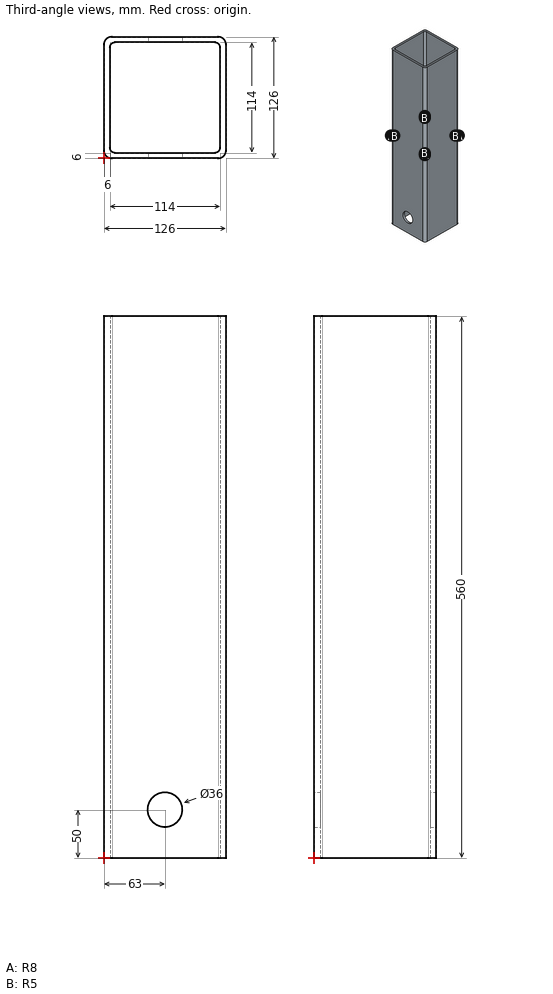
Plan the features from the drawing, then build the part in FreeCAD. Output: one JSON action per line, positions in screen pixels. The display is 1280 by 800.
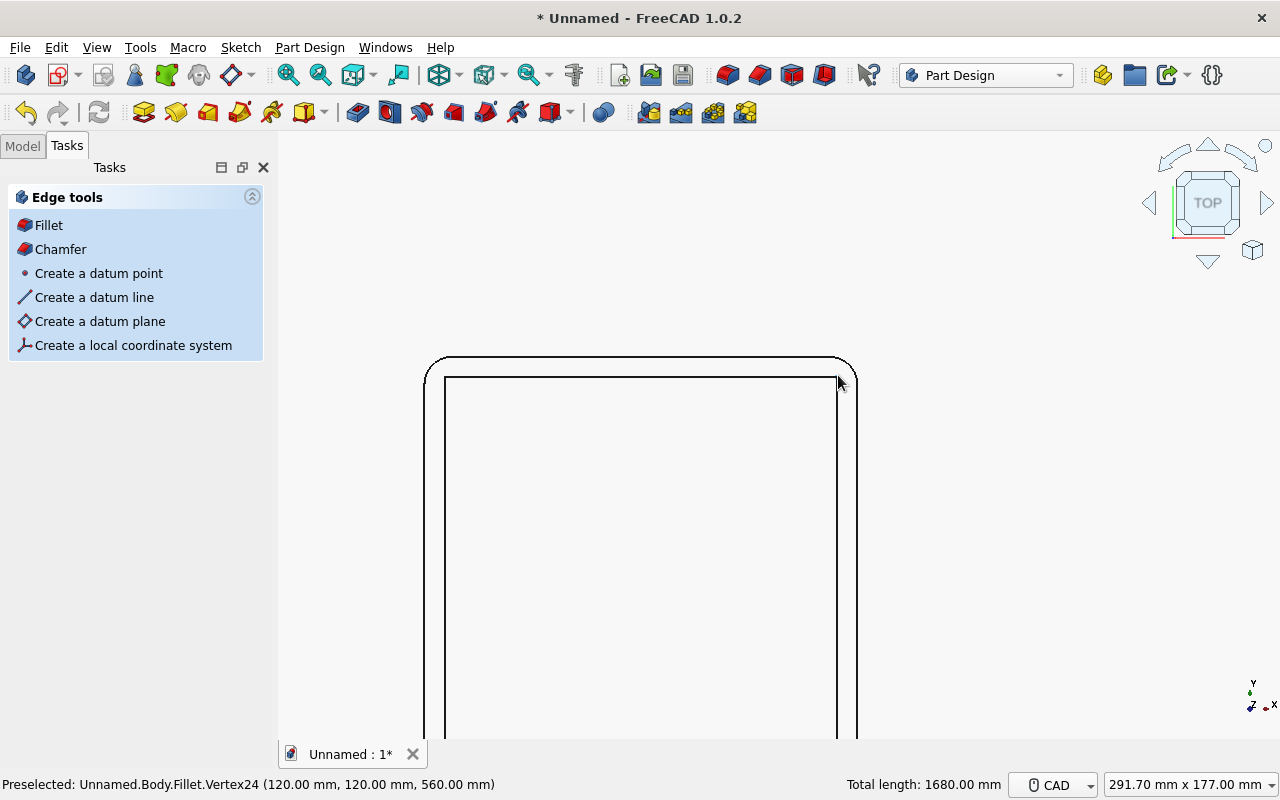
{"action": "left_click", "coordinate": [290, 76]}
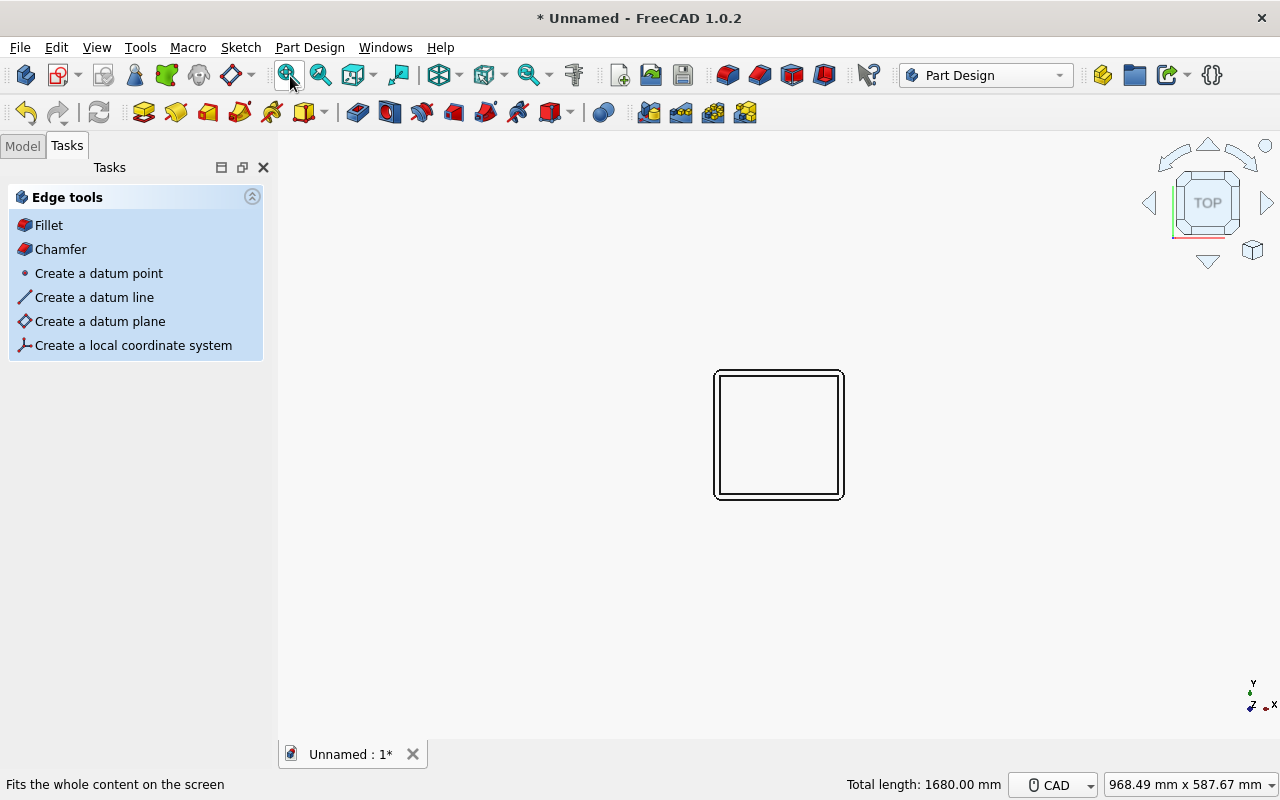
{"action": "key", "text": "1"}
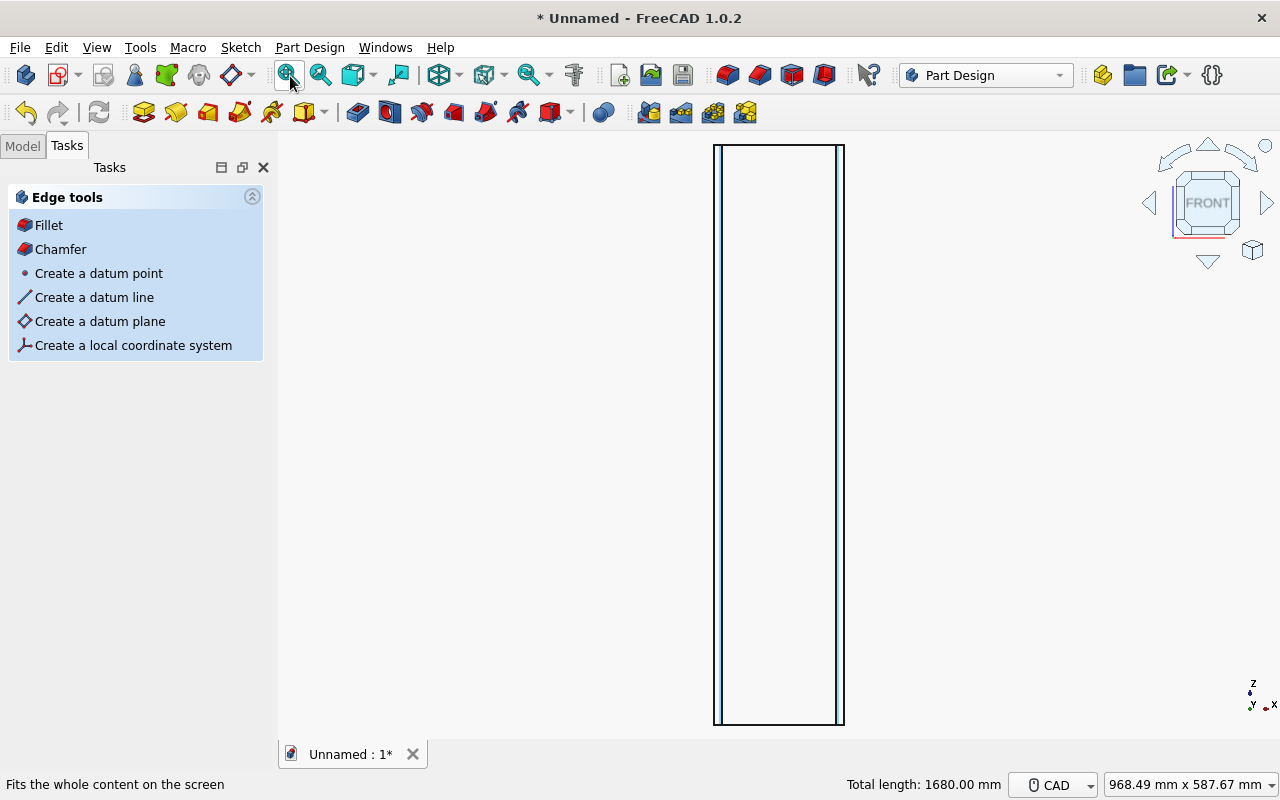
{"action": "scroll", "coordinate": [838, 434], "scroll_direction": "up", "scroll_amount": 6}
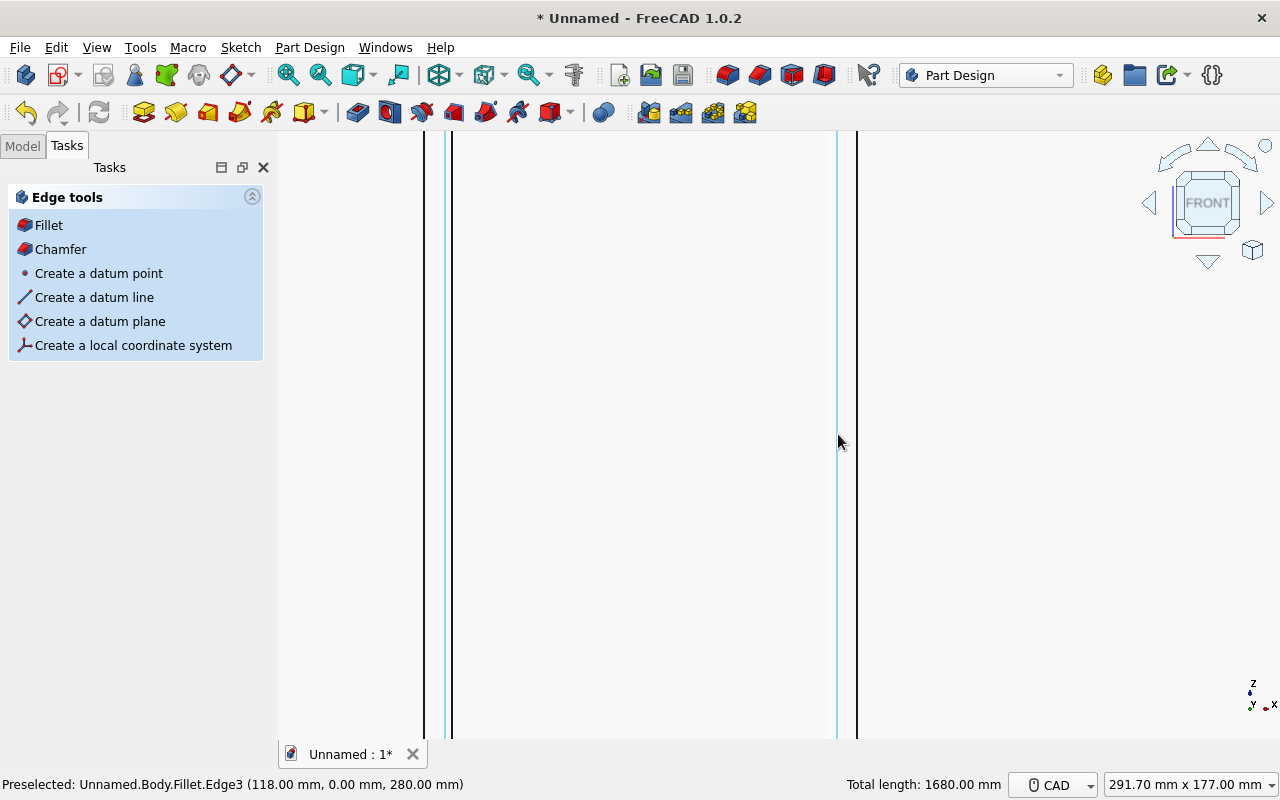
{"action": "left_click", "coordinate": [290, 76]}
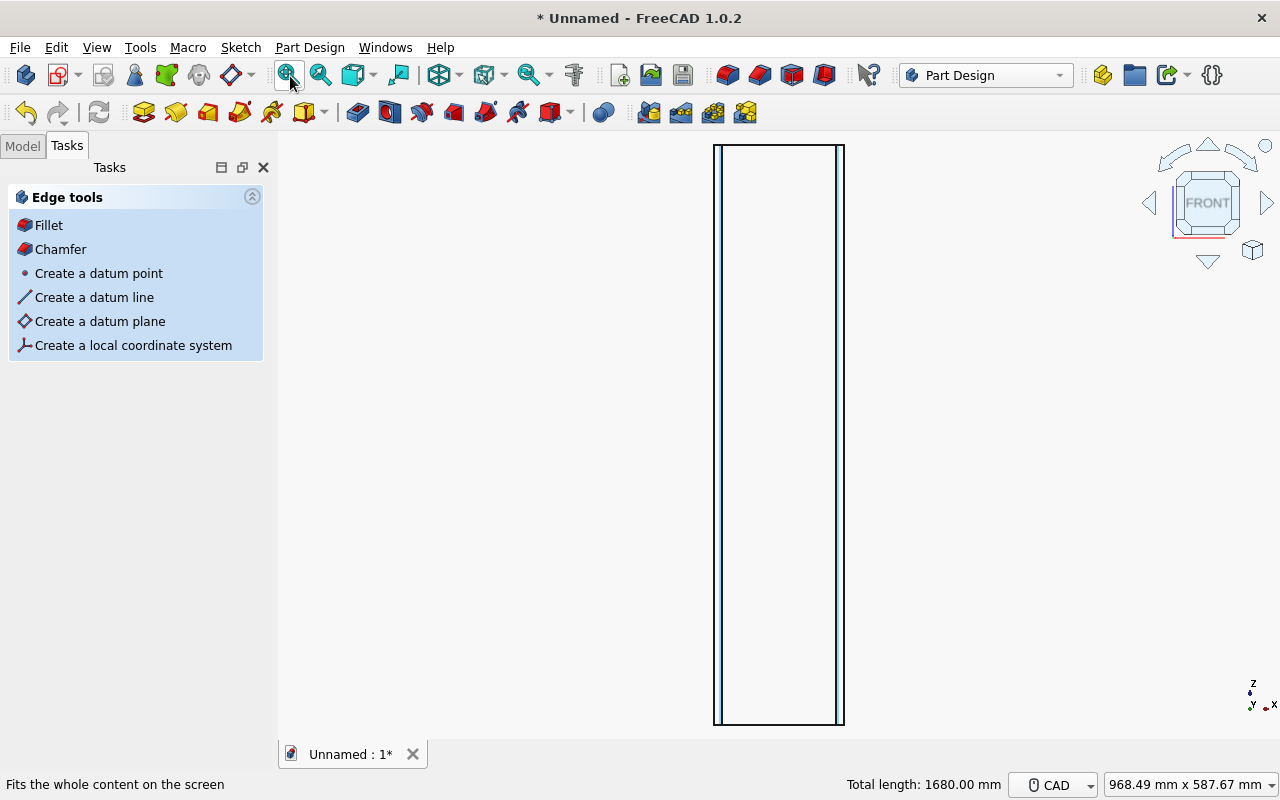
{"action": "key", "text": "3"}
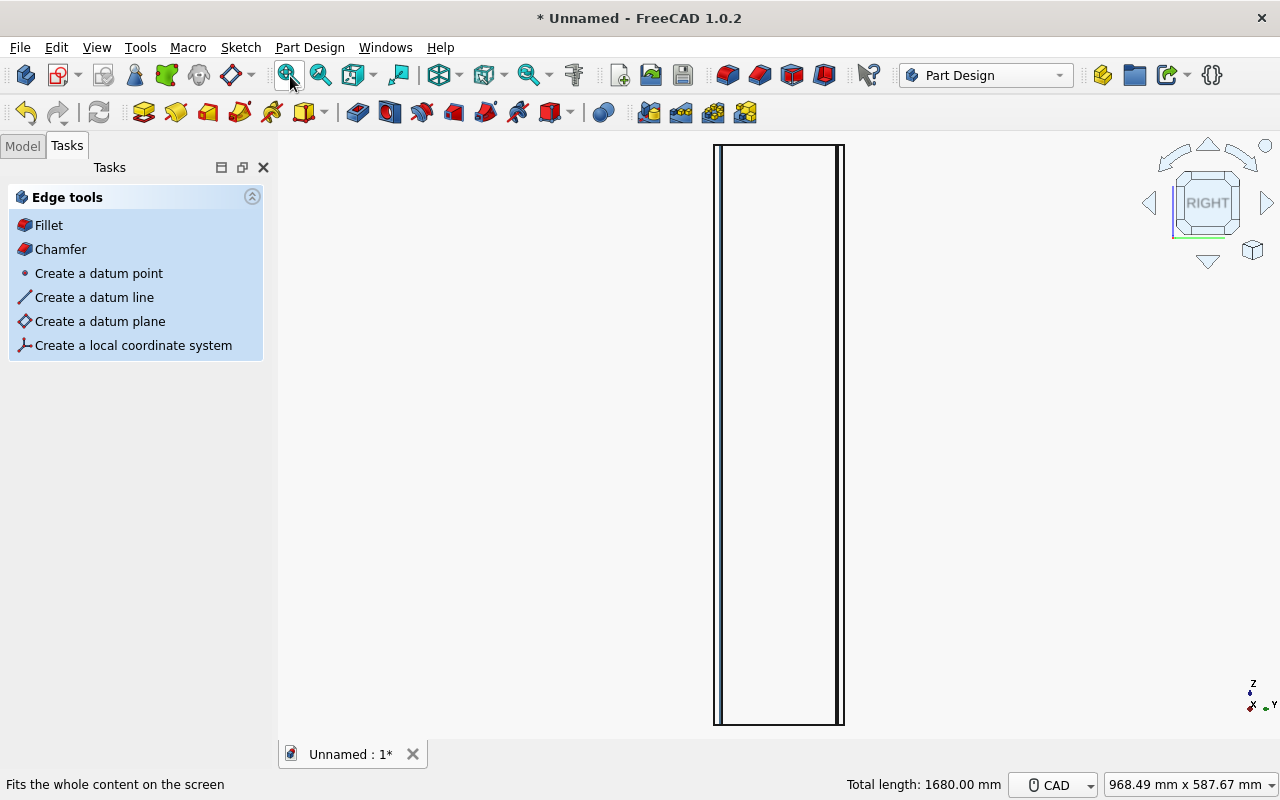
{"action": "scroll", "coordinate": [838, 434], "scroll_direction": "up", "scroll_amount": 6}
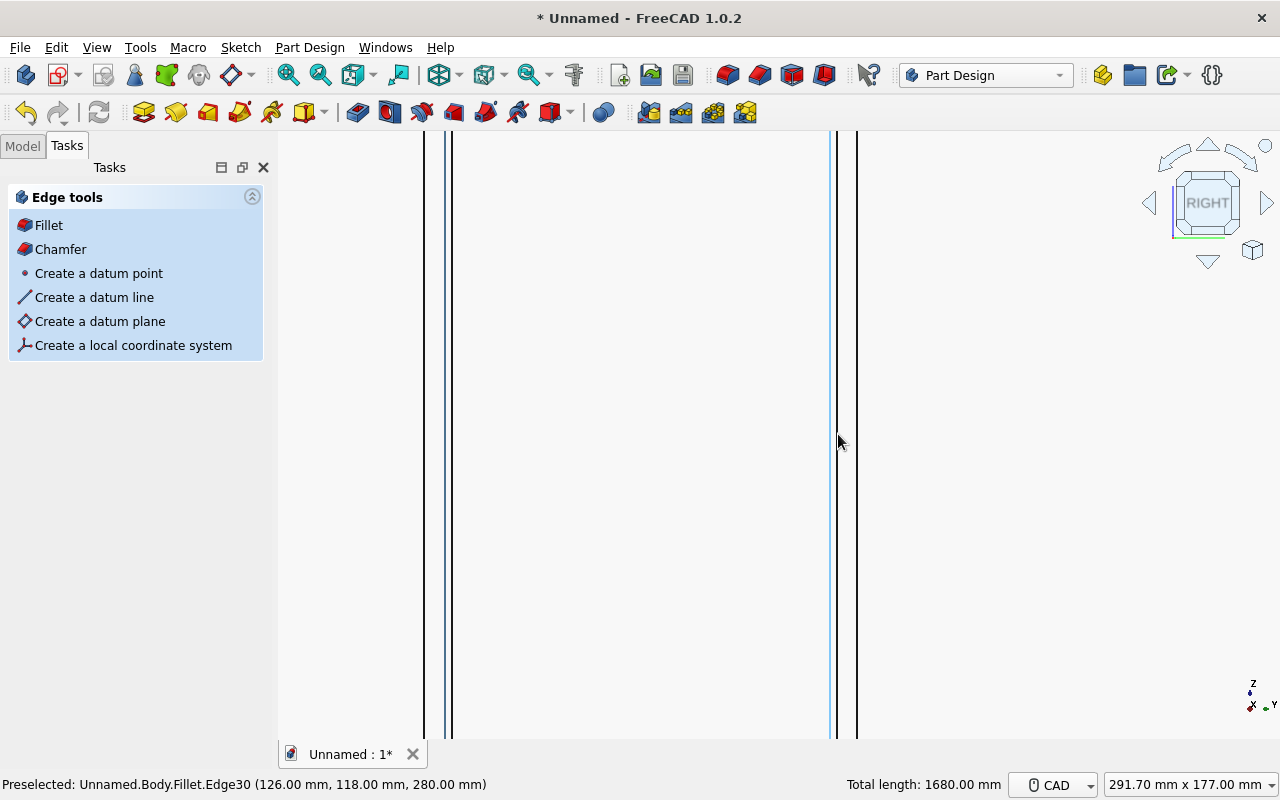
{"action": "left_click", "coordinate": [837, 435], "text": "ctrl"}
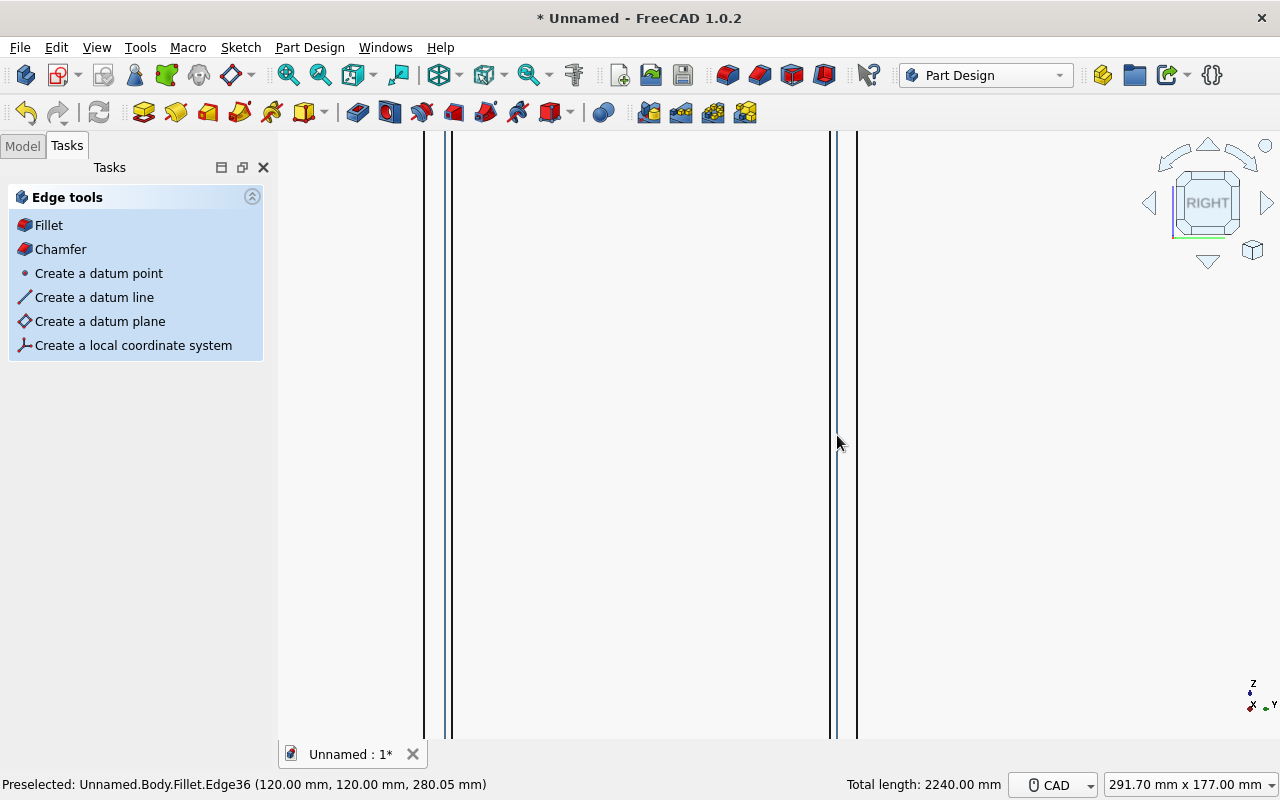
{"action": "key", "text": "v 1"}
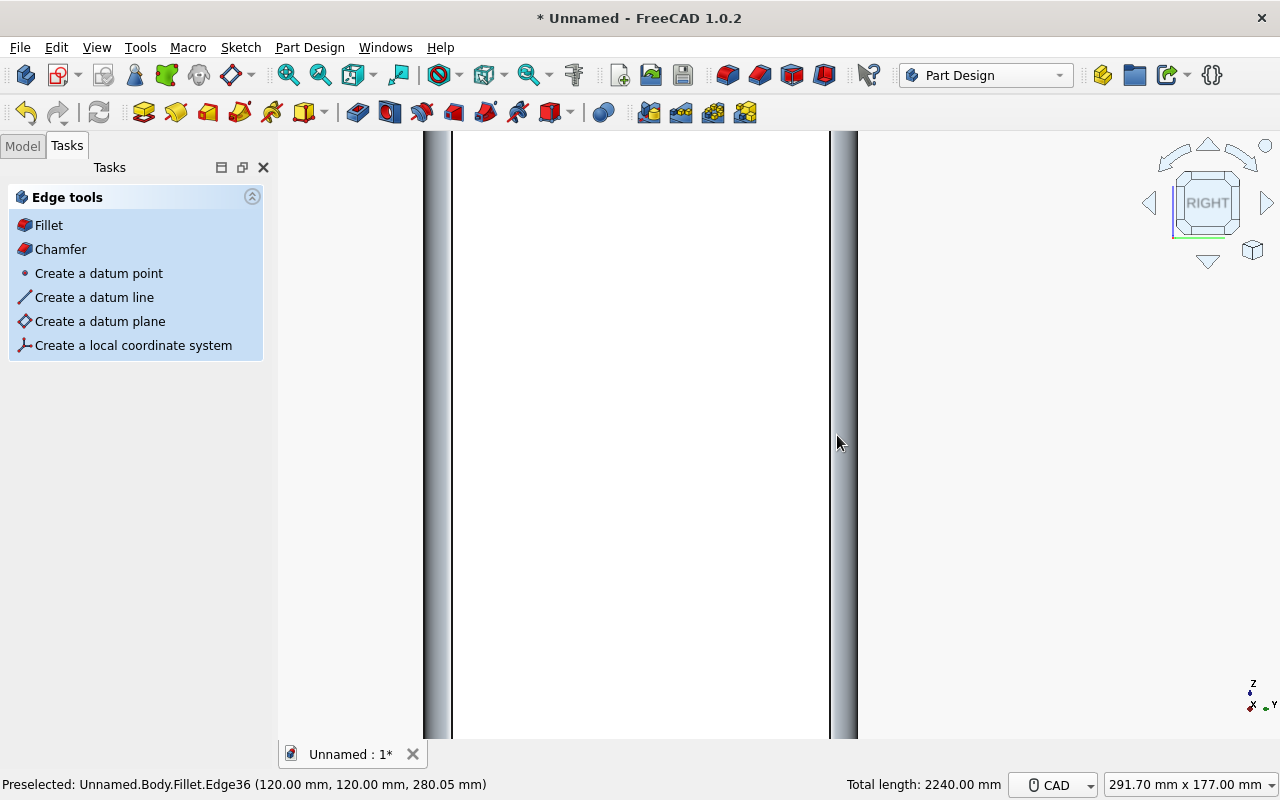
{"action": "left_click", "coordinate": [728, 76]}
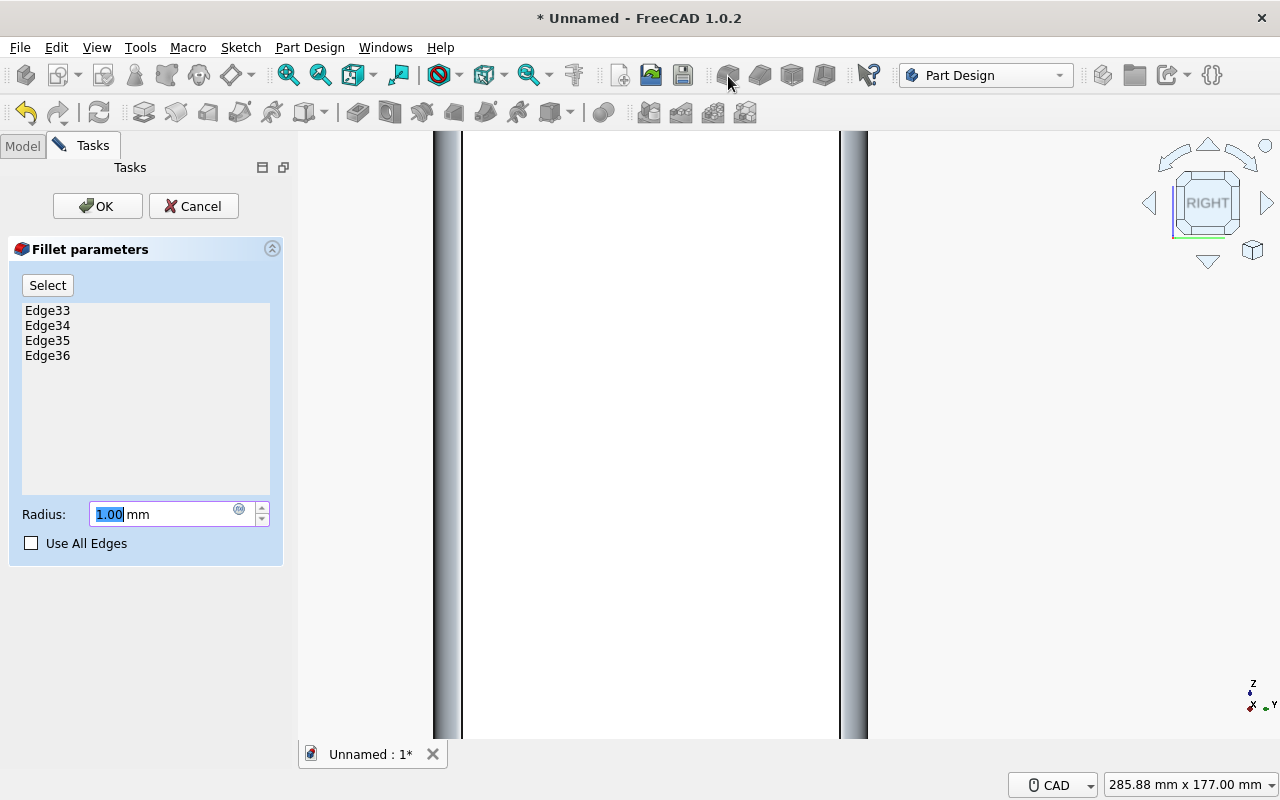
{"action": "type", "text": "5"}
{"action": "key", "text": "Tab"}